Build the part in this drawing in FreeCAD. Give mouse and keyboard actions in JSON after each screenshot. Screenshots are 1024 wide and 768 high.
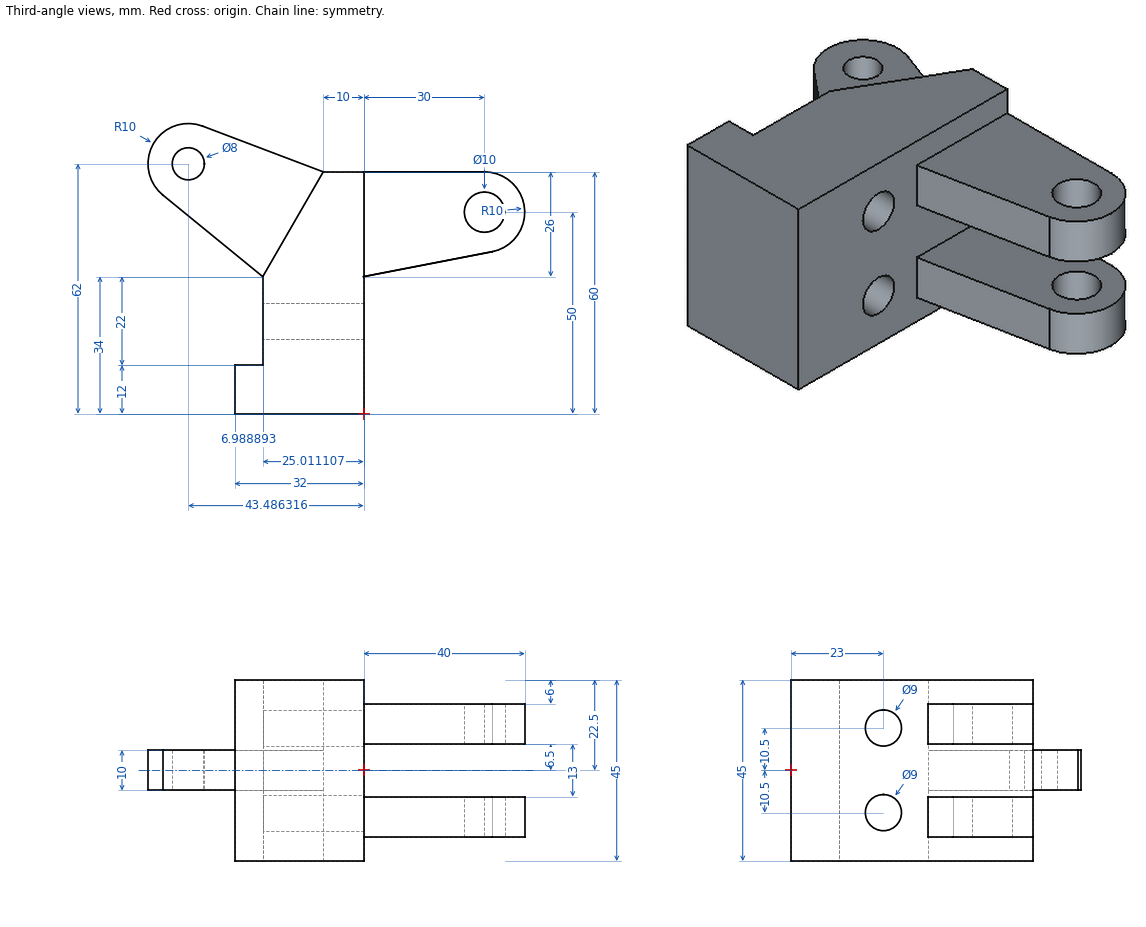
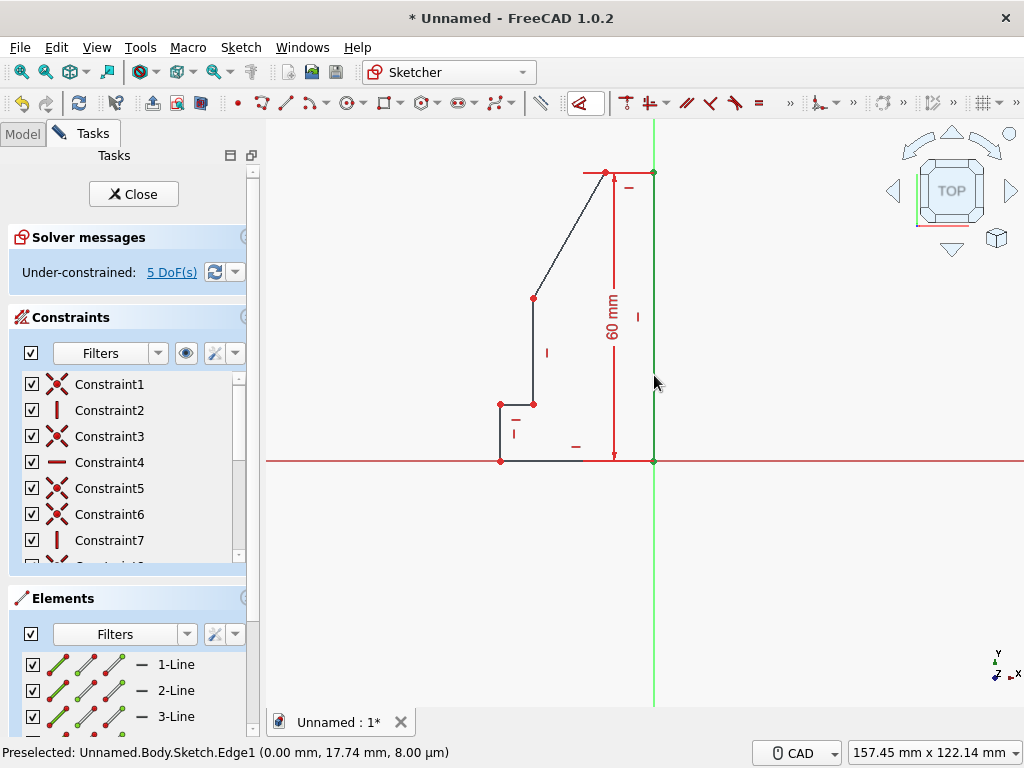
{"action": "left_click", "coordinate": [639, 173]}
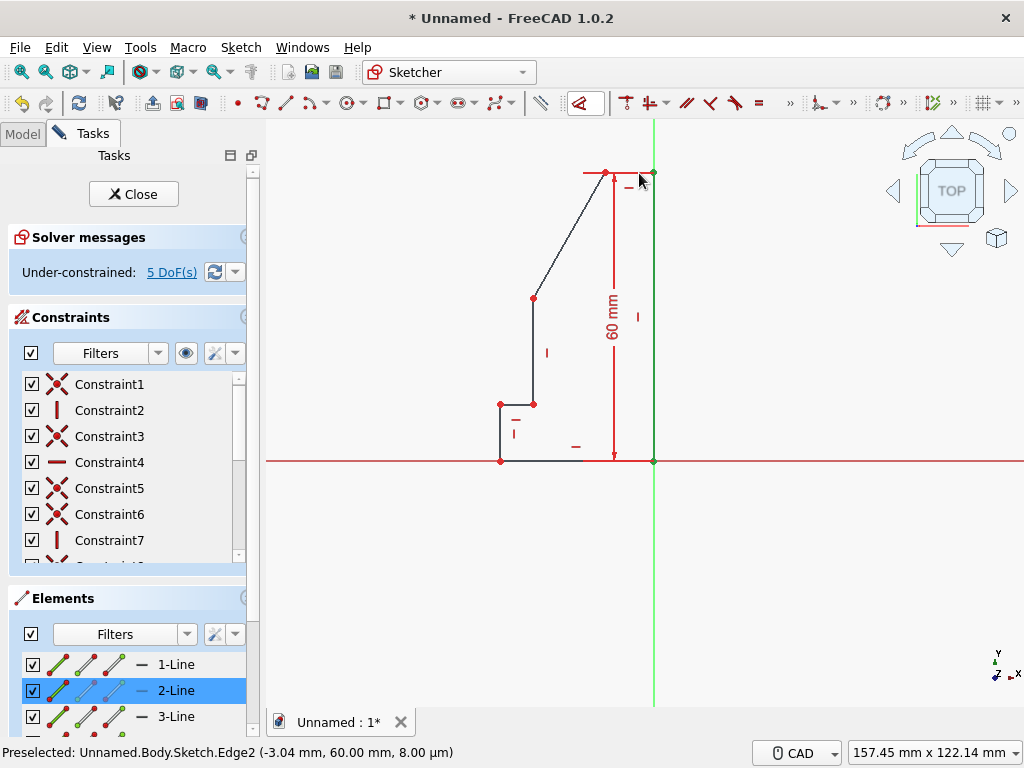
{"action": "key", "text": "l"}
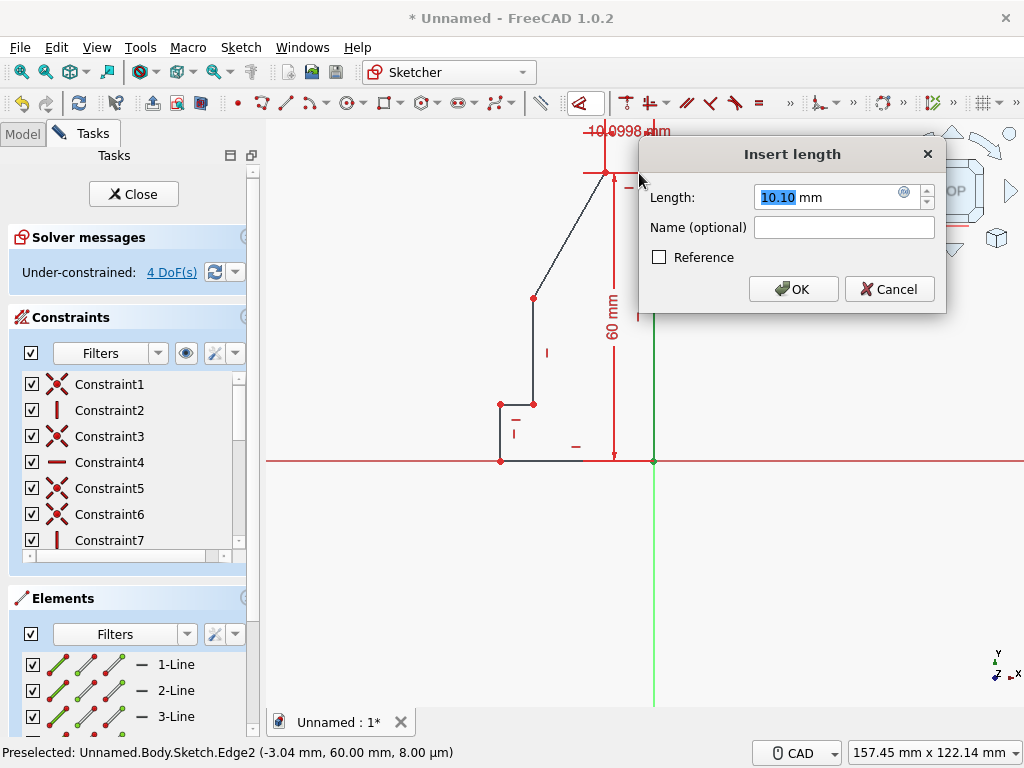
{"action": "type", "text": "10"}
{"action": "key", "text": "Return"}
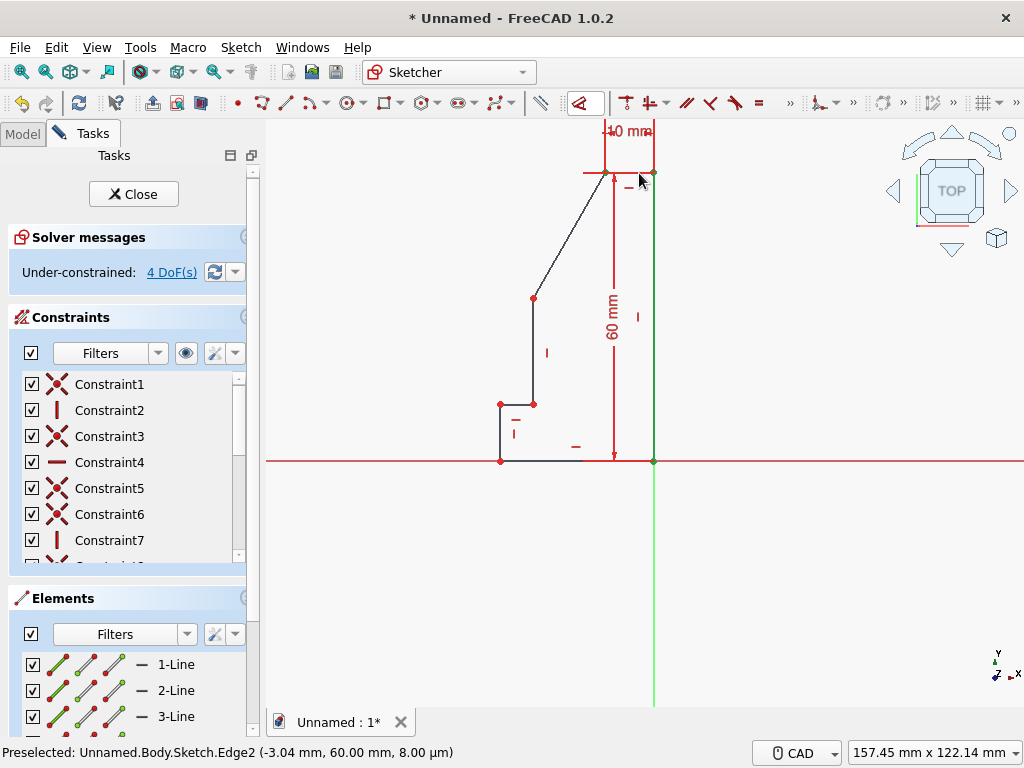
{"action": "left_click", "coordinate": [533, 331]}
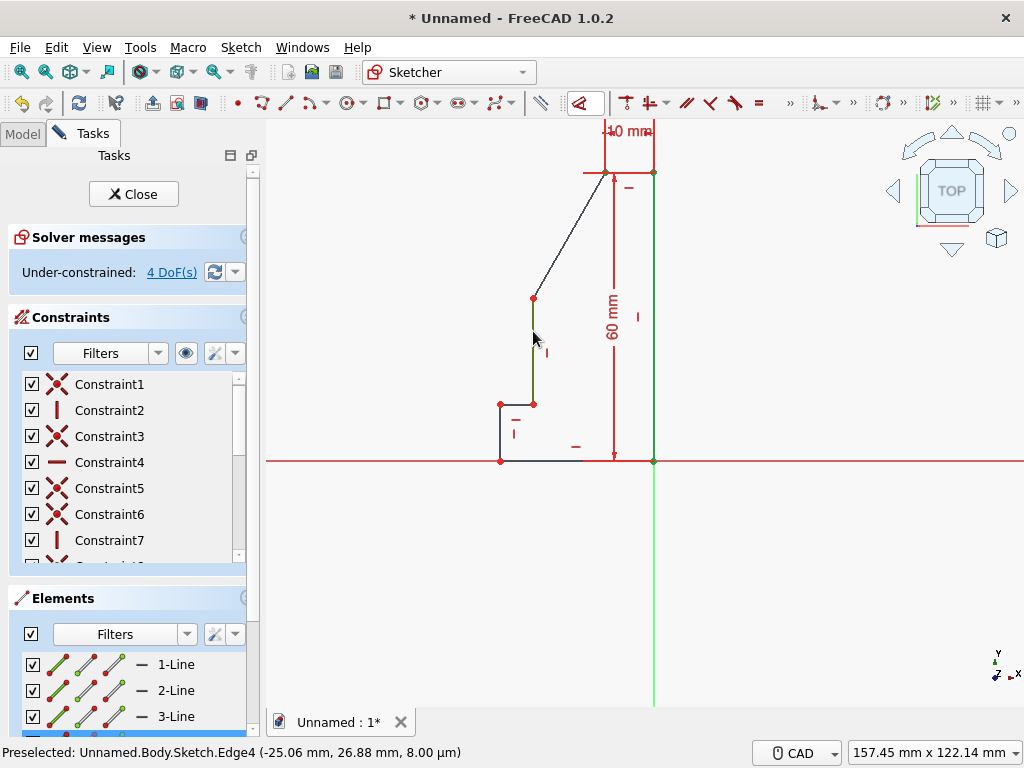
{"action": "left_click", "coordinate": [598, 104]}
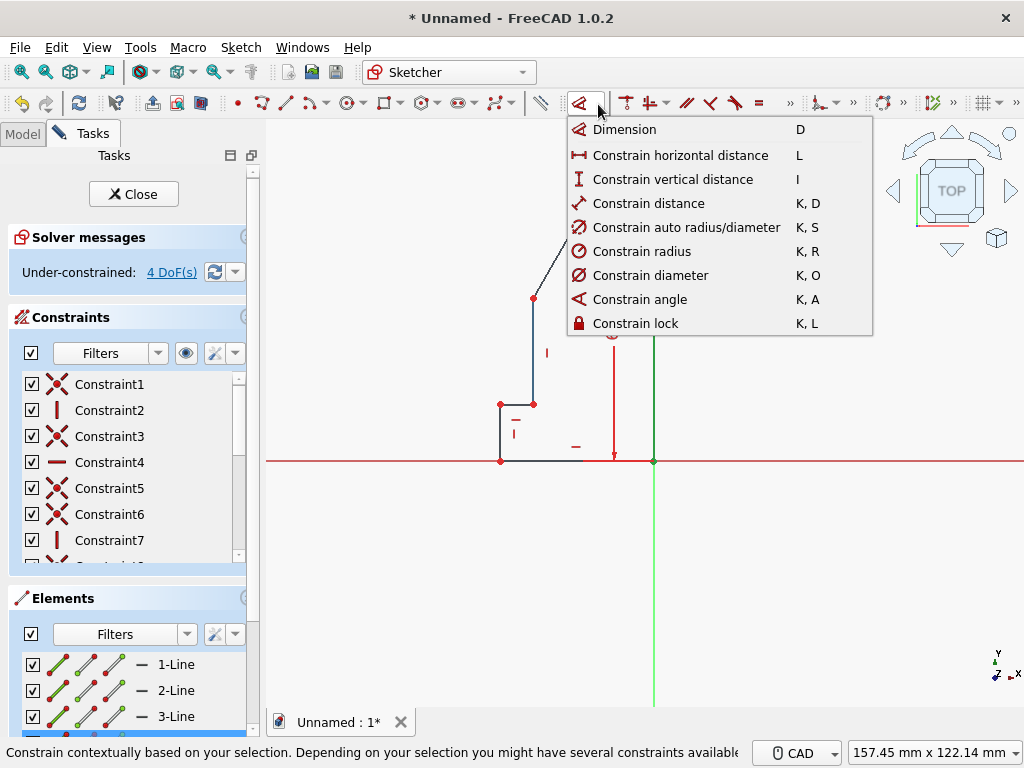
{"action": "left_click", "coordinate": [720, 179]}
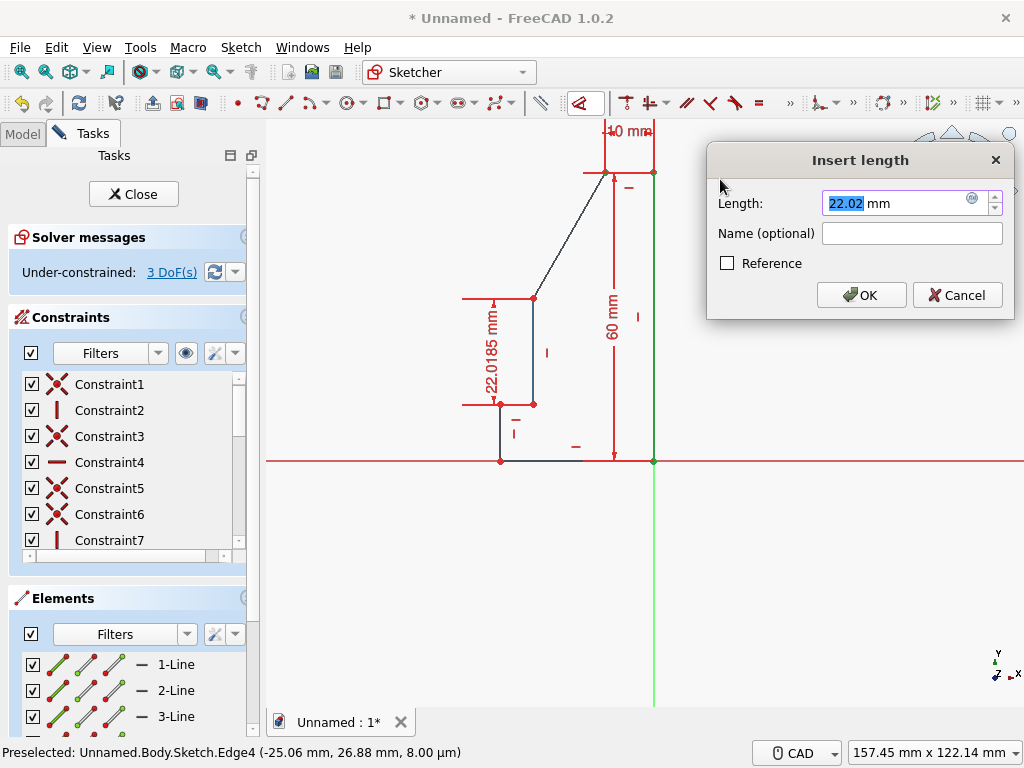
{"action": "type", "text": "22"}
{"action": "key", "text": "Return"}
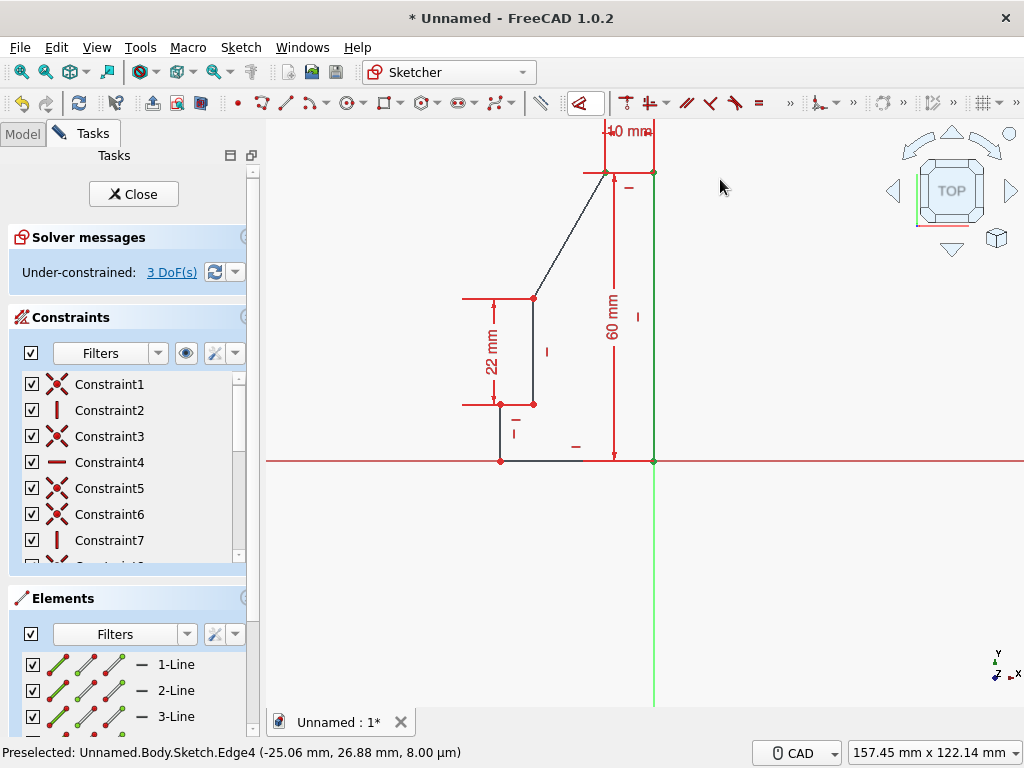
{"action": "left_click", "coordinate": [500, 422]}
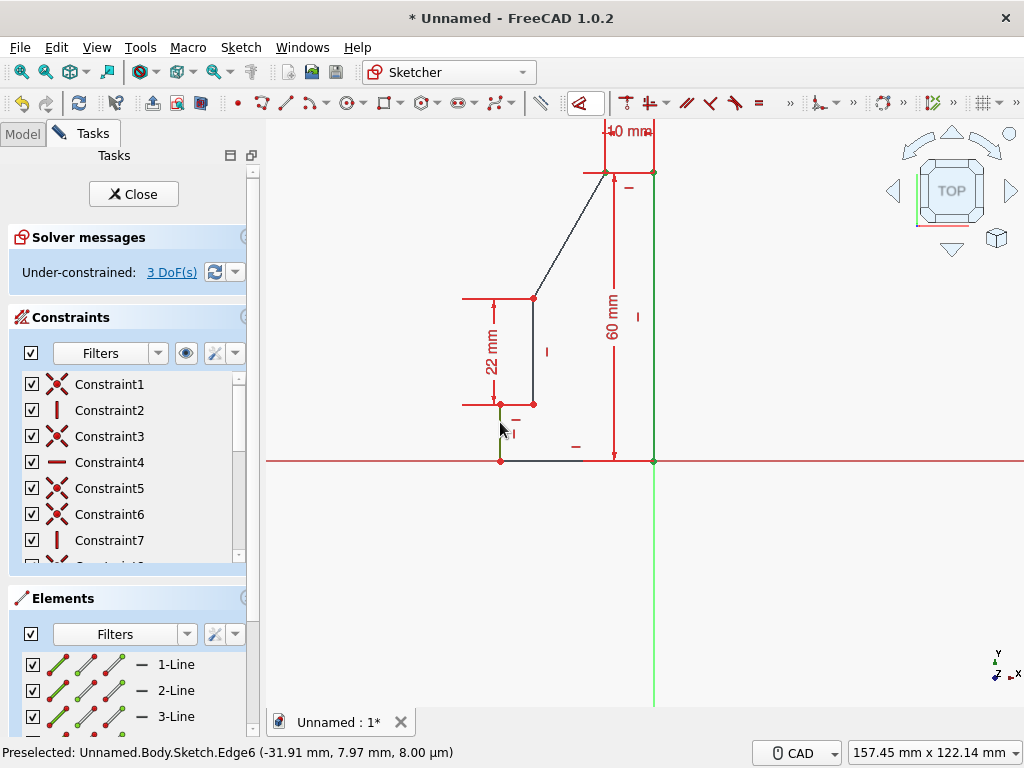
{"action": "key", "text": "i"}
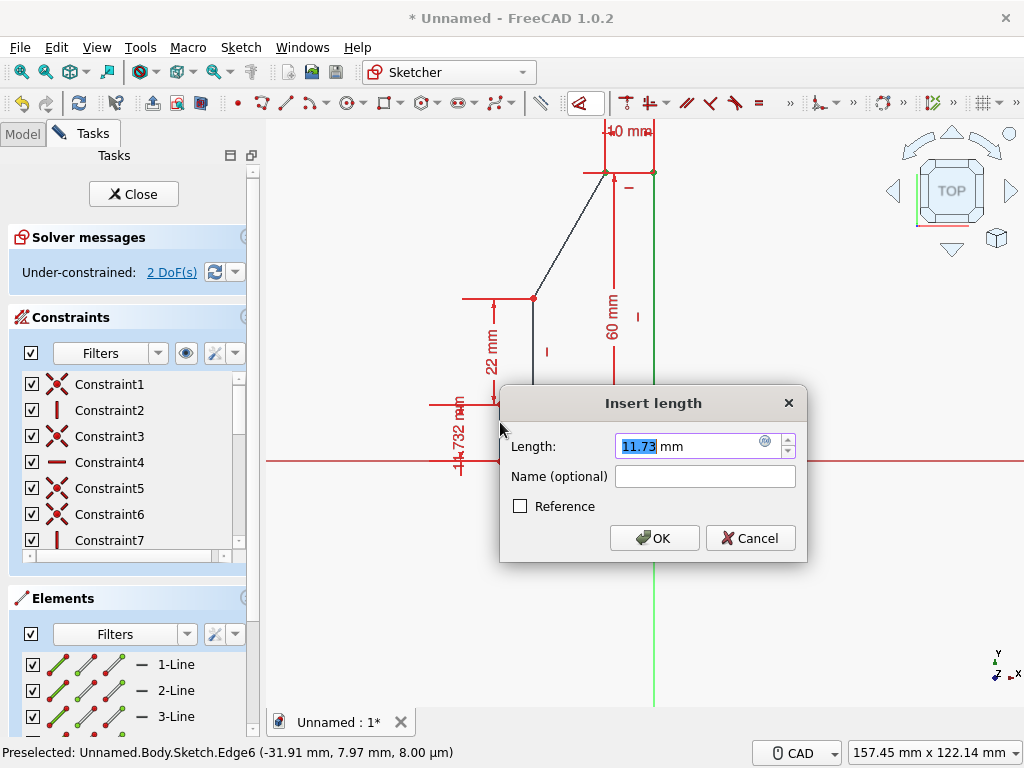
{"action": "type", "text": "12"}
{"action": "key", "text": "Return"}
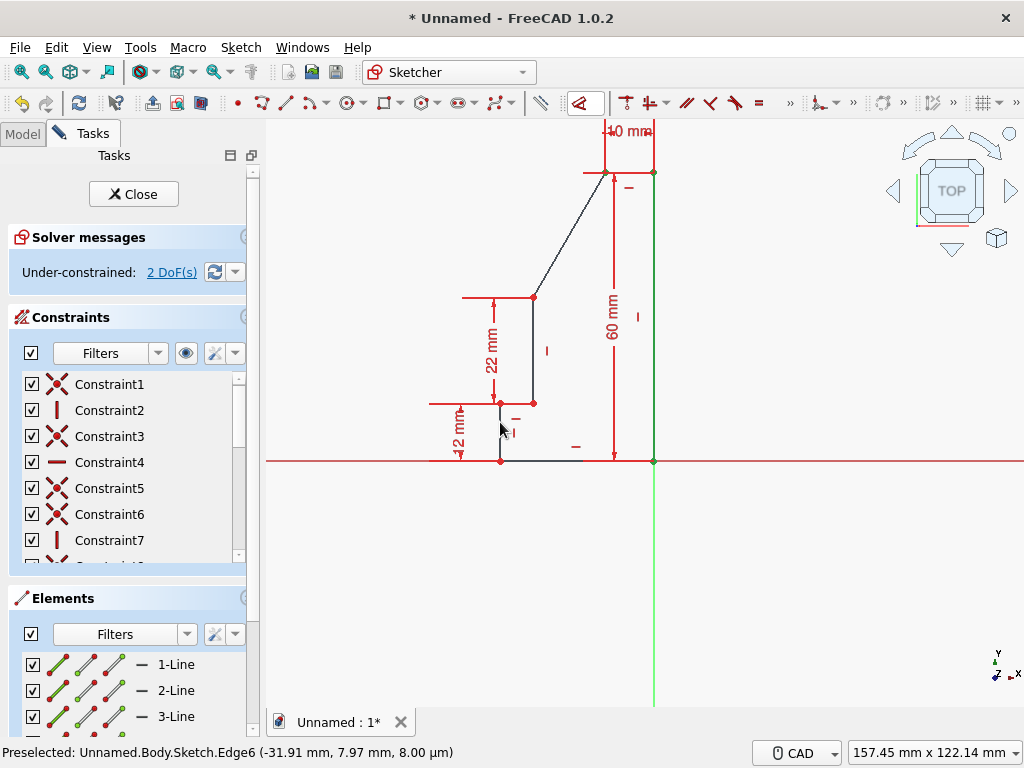
{"action": "left_click", "coordinate": [546, 461]}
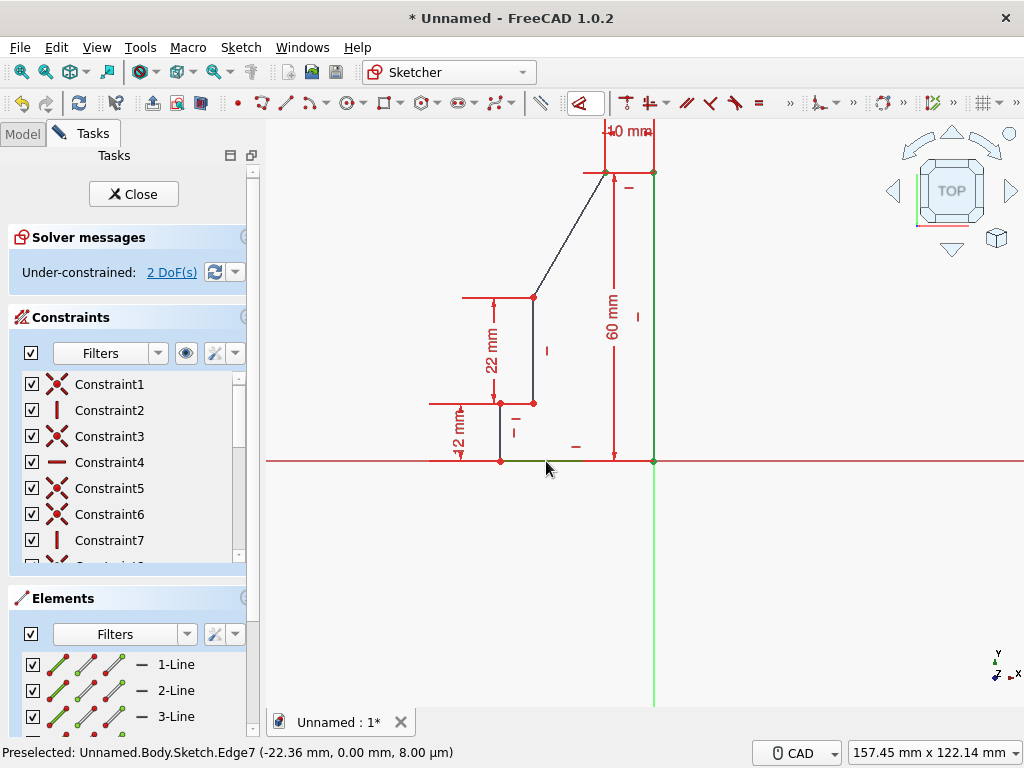
{"action": "left_click", "coordinate": [598, 104]}